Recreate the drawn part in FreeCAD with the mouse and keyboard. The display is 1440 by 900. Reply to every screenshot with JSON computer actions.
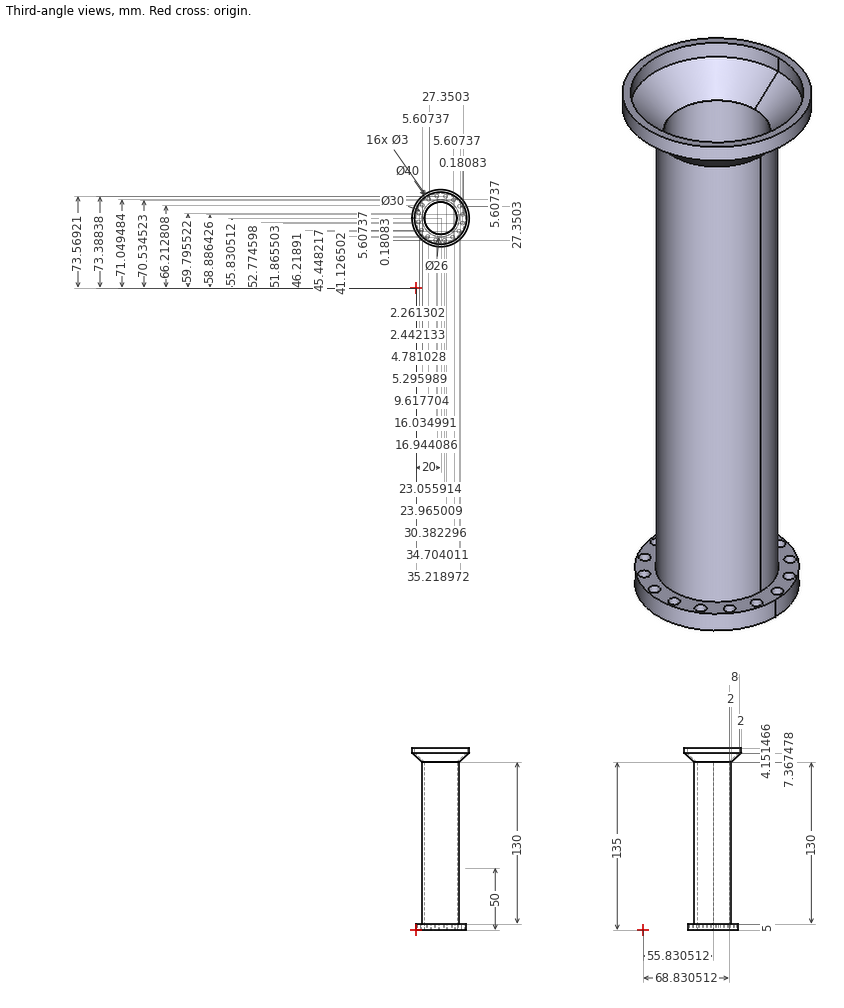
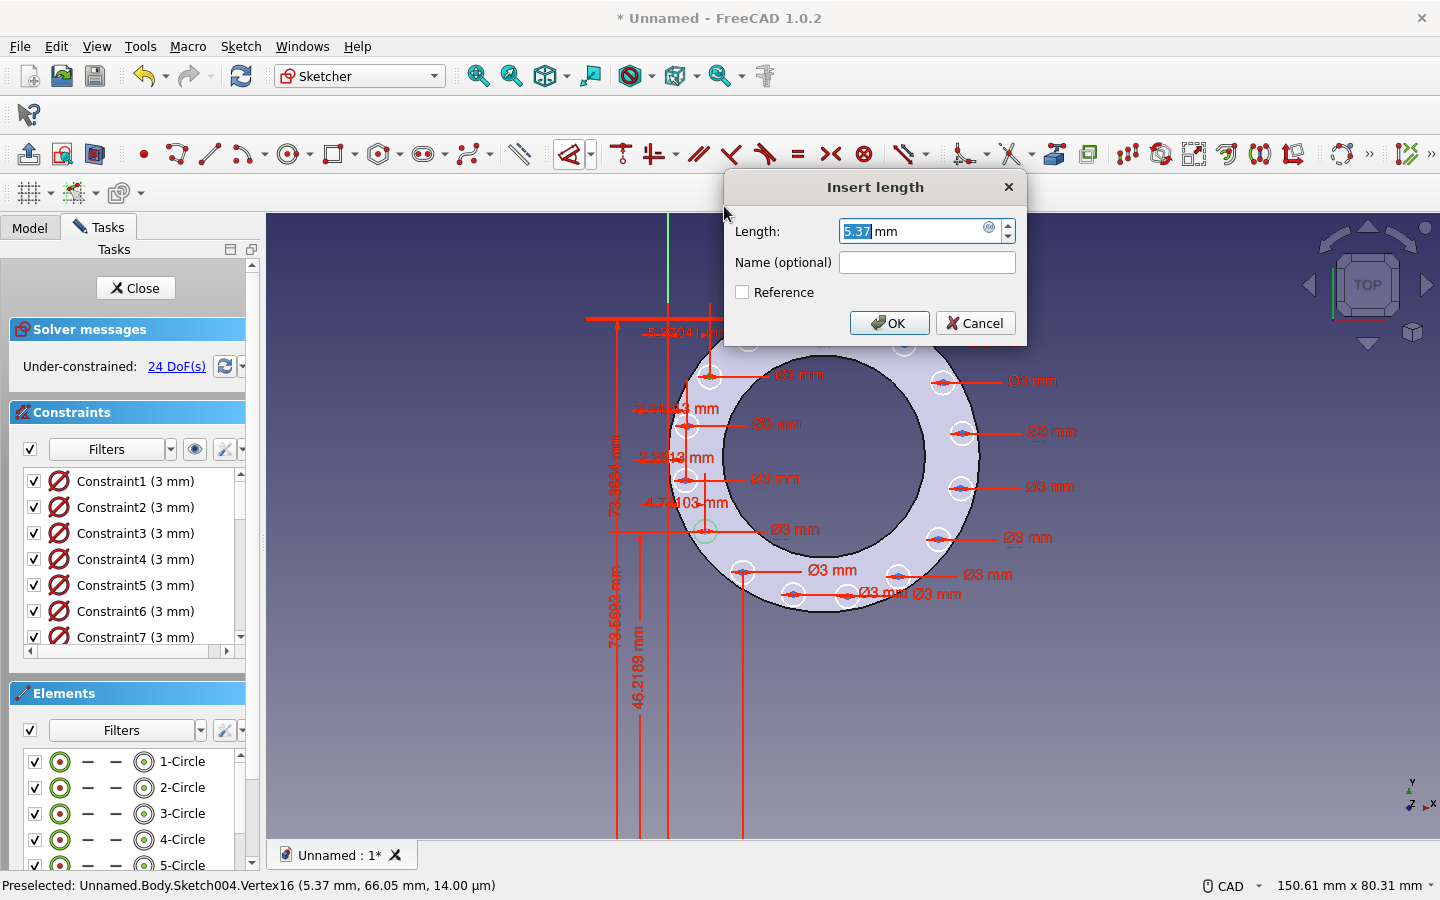
{"action": "type", "text": "5.295989"}
{"action": "key", "text": "Return"}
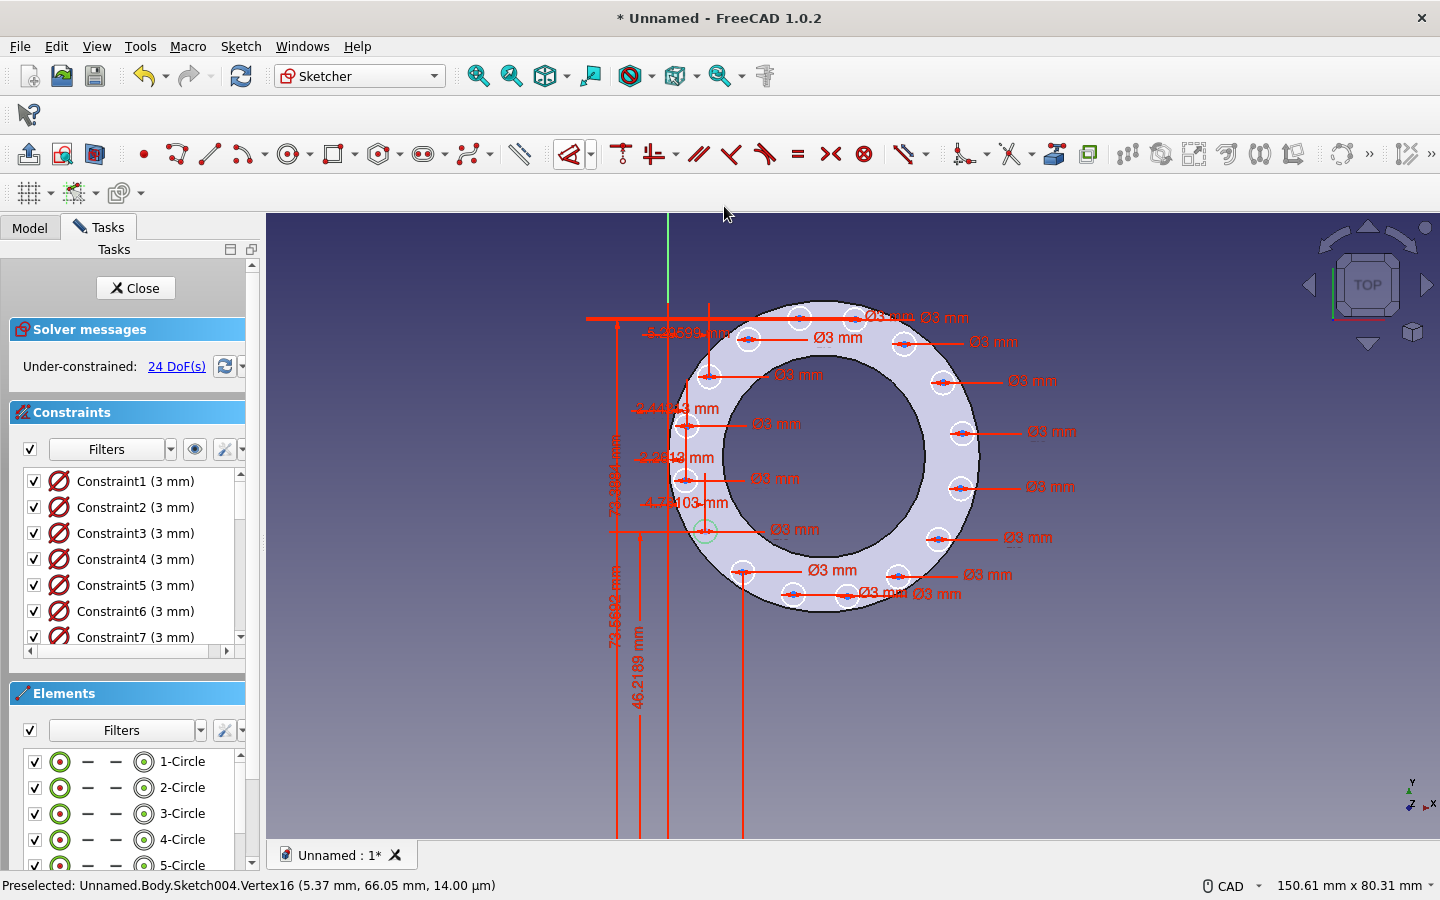
{"action": "left_click", "coordinate": [749, 340]}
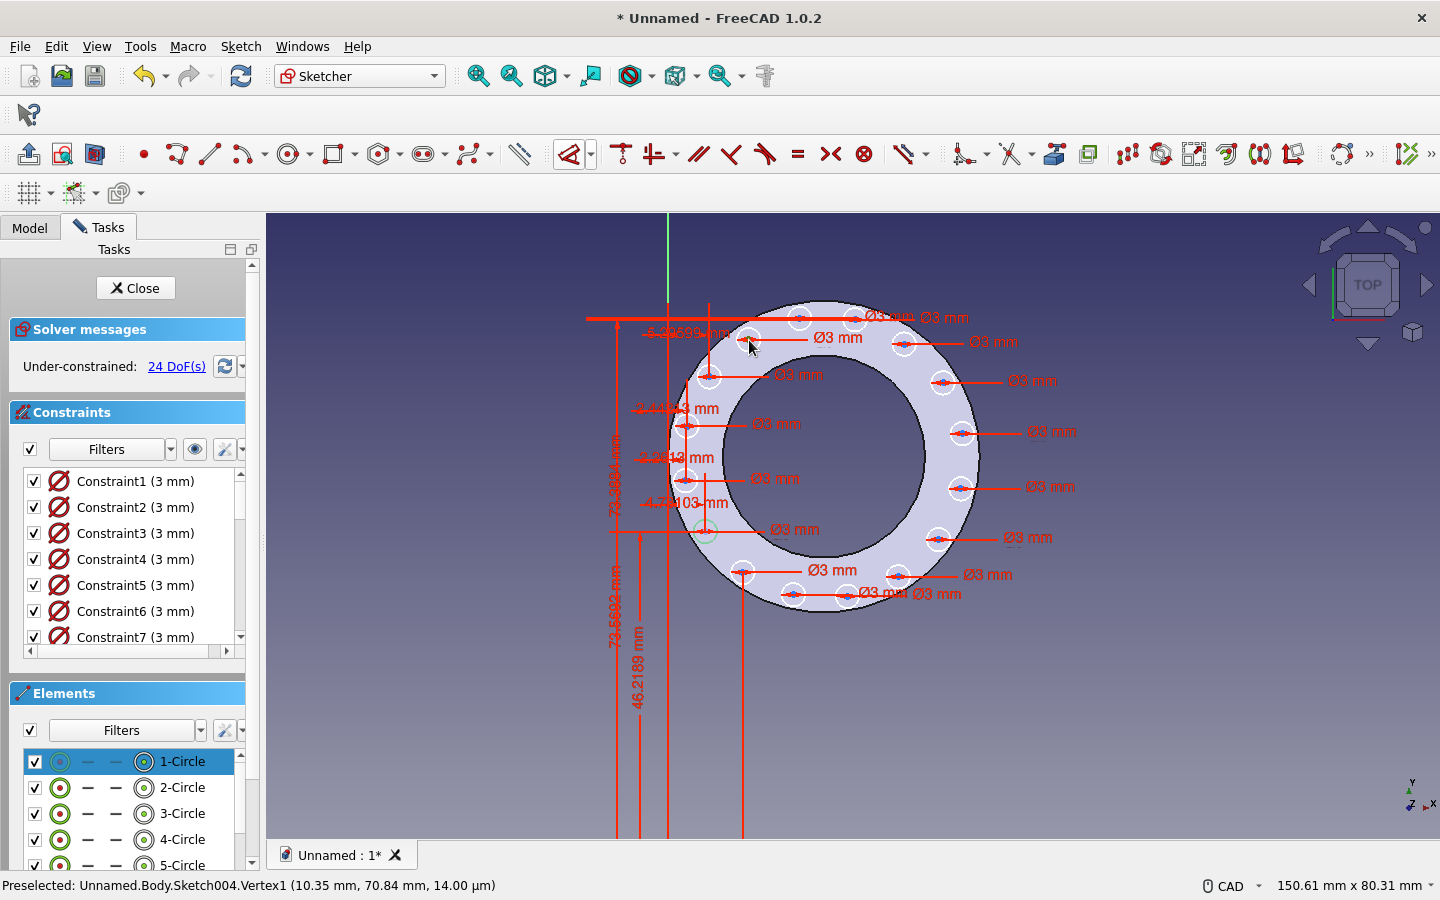
{"action": "left_click", "coordinate": [943, 383]}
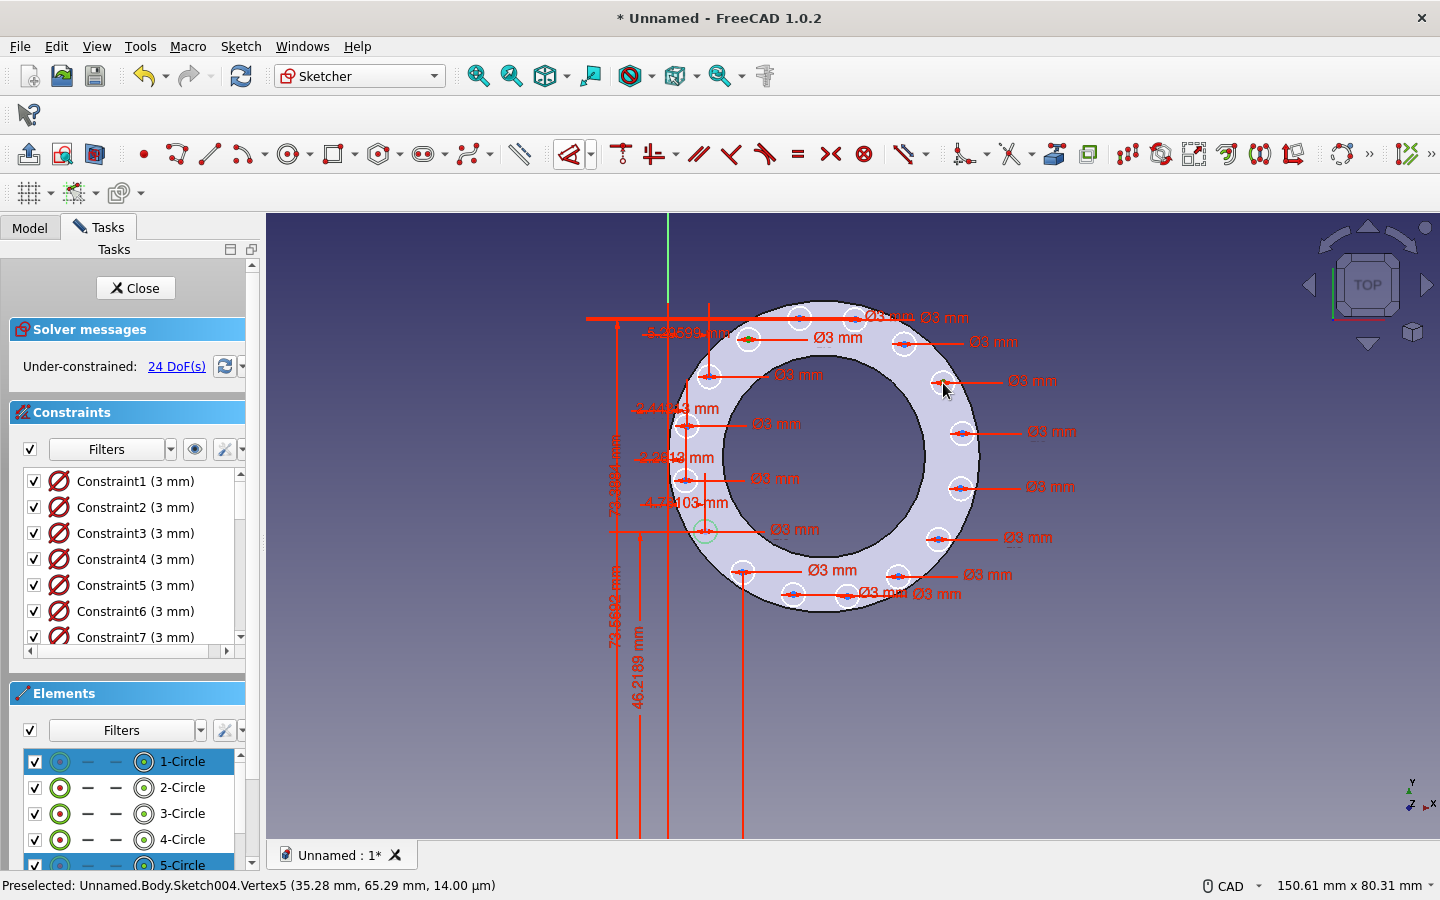
{"action": "left_click", "coordinate": [590, 154]}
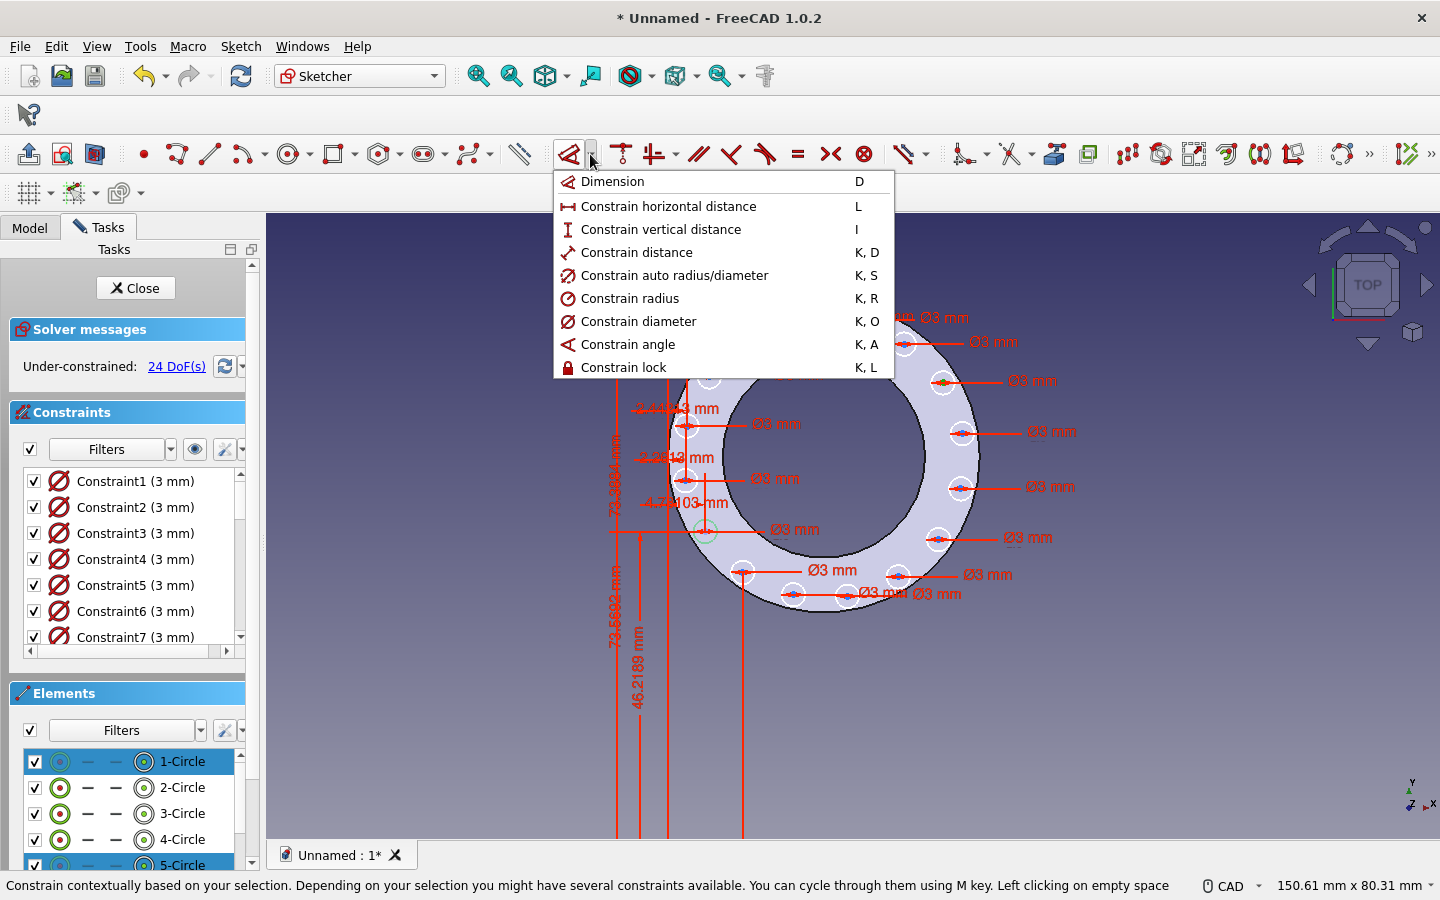
{"action": "left_click", "coordinate": [724, 230]}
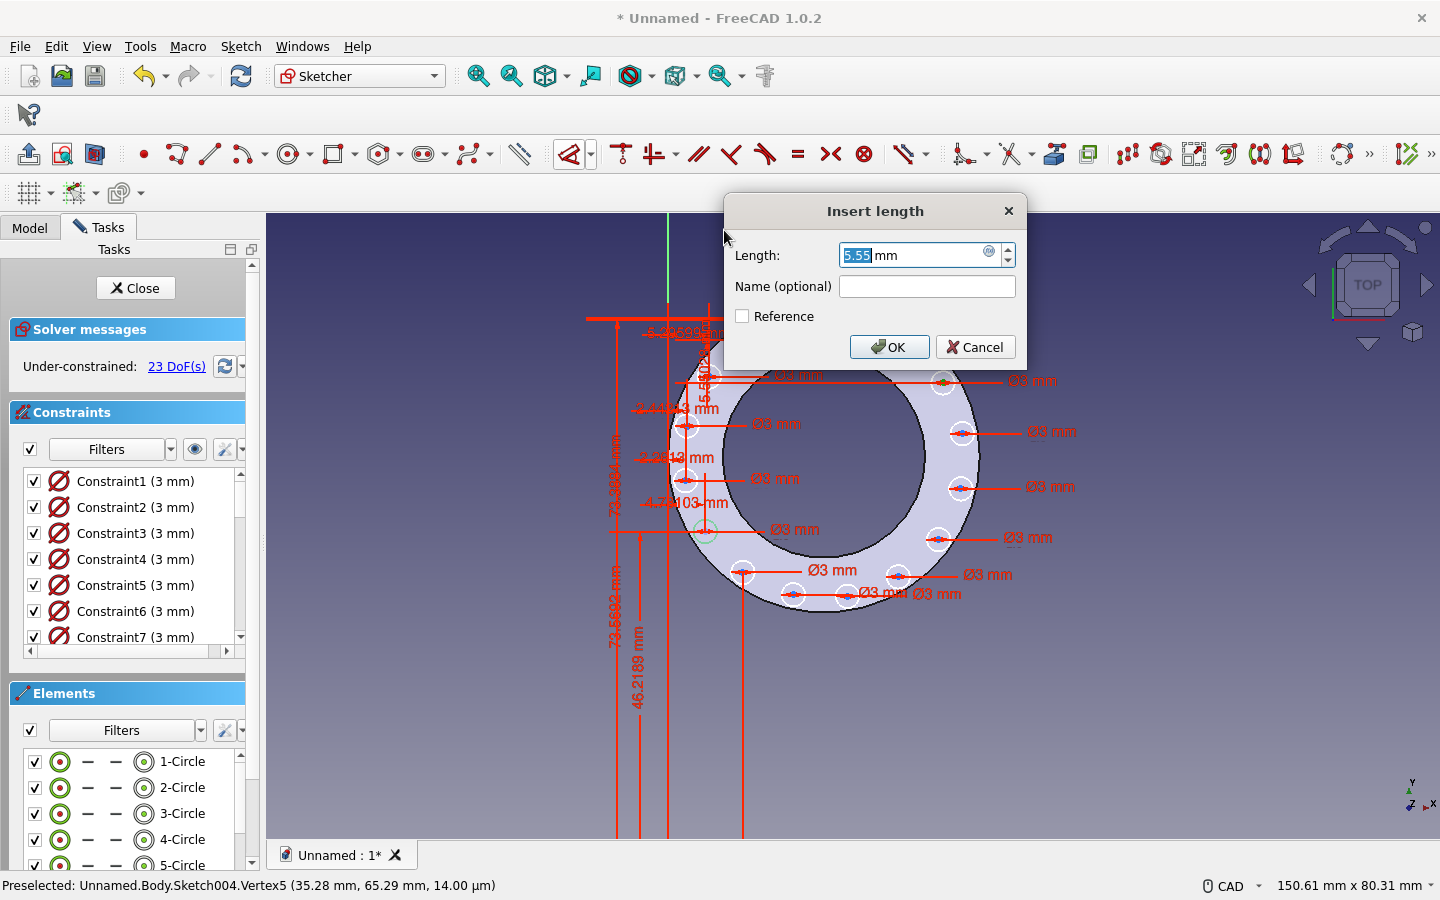
{"action": "type", "text": "5.60737"}
{"action": "key", "text": "Return"}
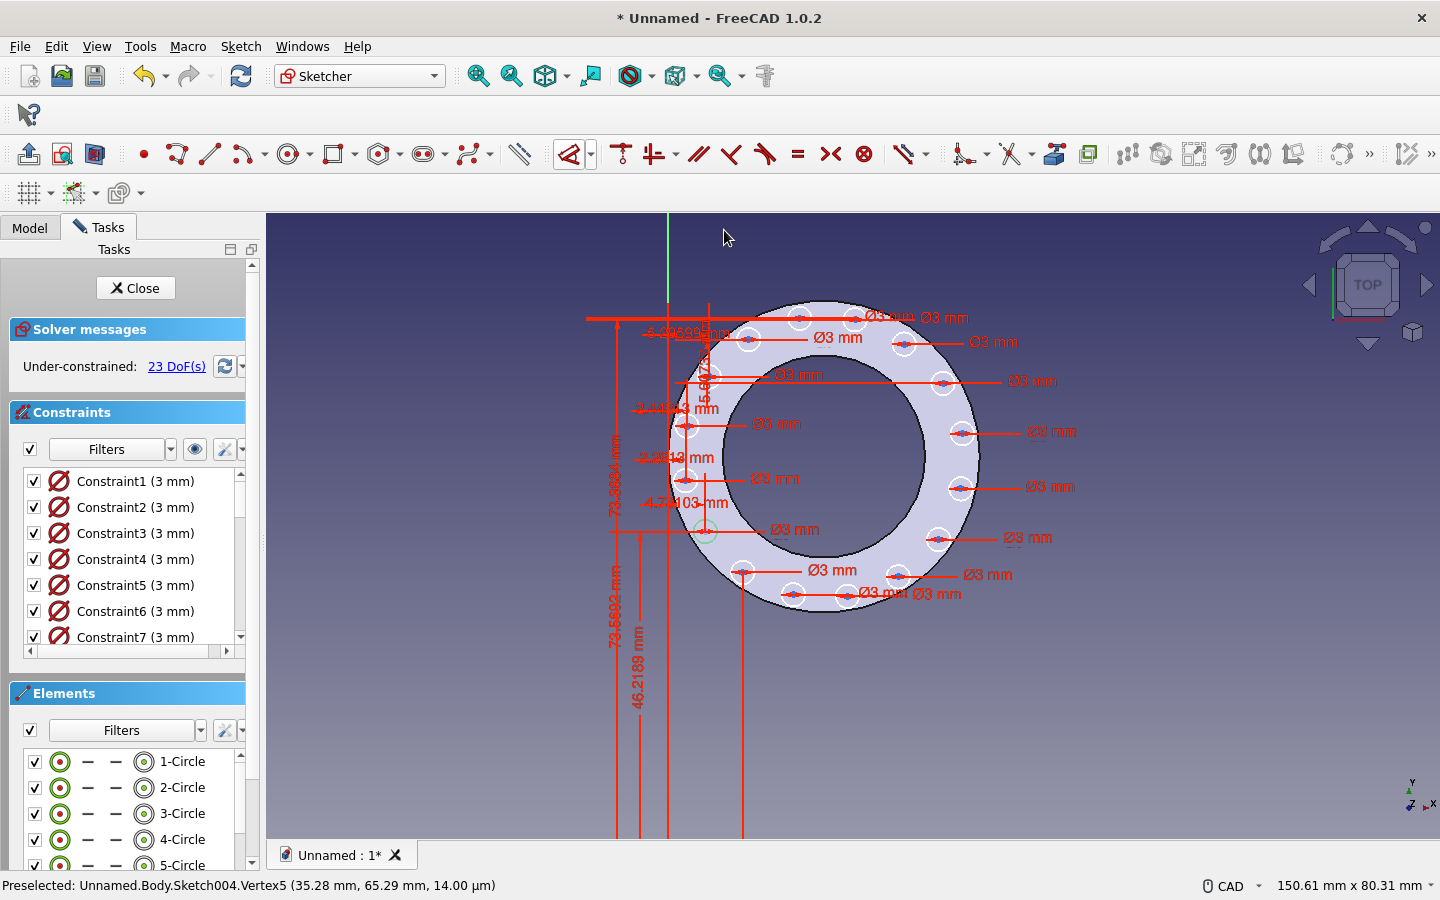
{"action": "left_click", "coordinate": [749, 340]}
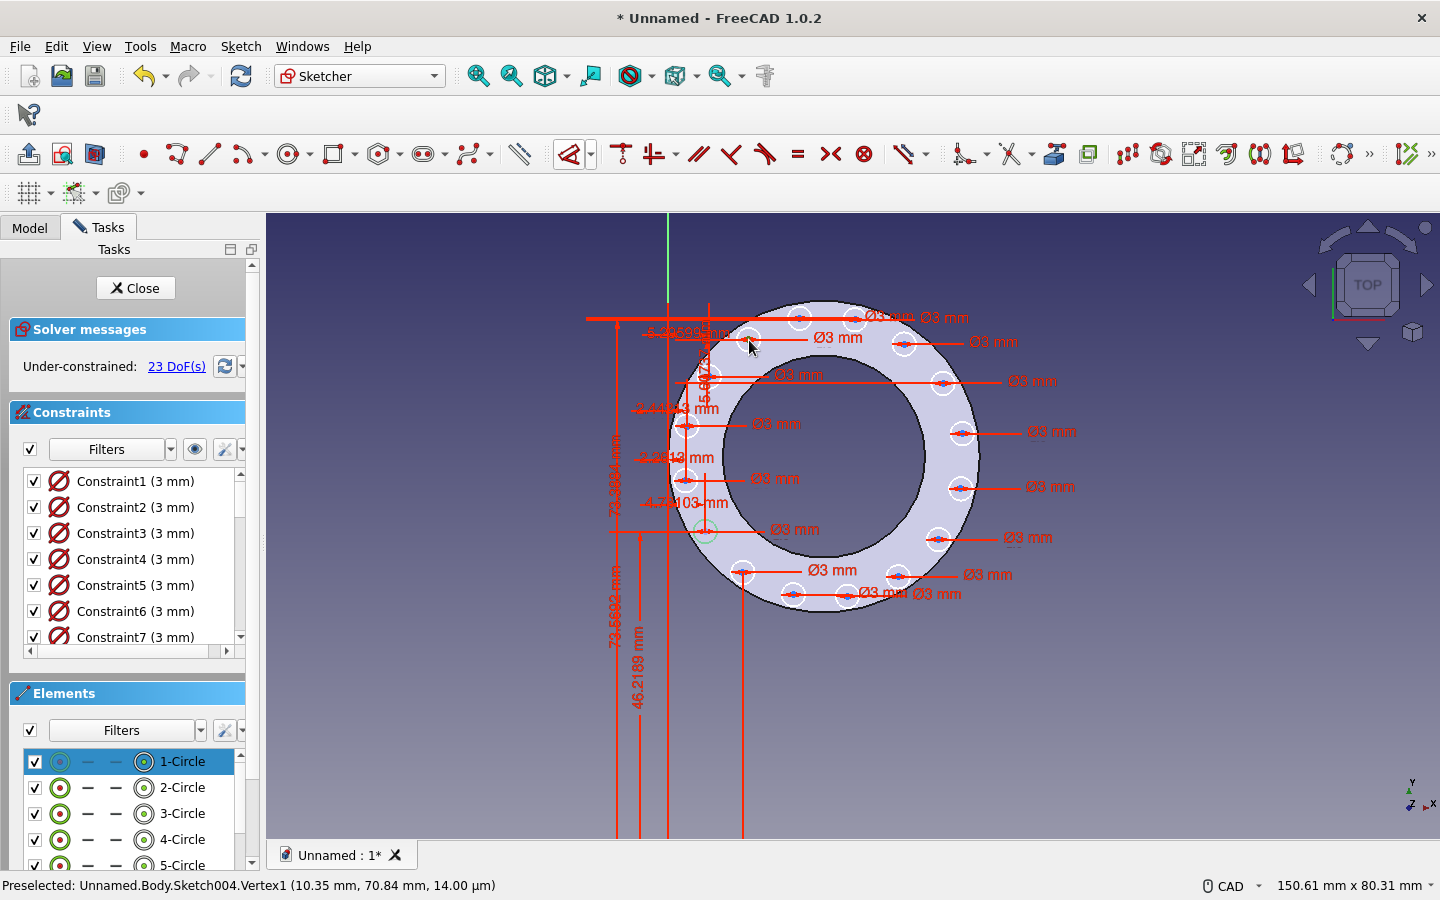
{"action": "left_click", "coordinate": [962, 434]}